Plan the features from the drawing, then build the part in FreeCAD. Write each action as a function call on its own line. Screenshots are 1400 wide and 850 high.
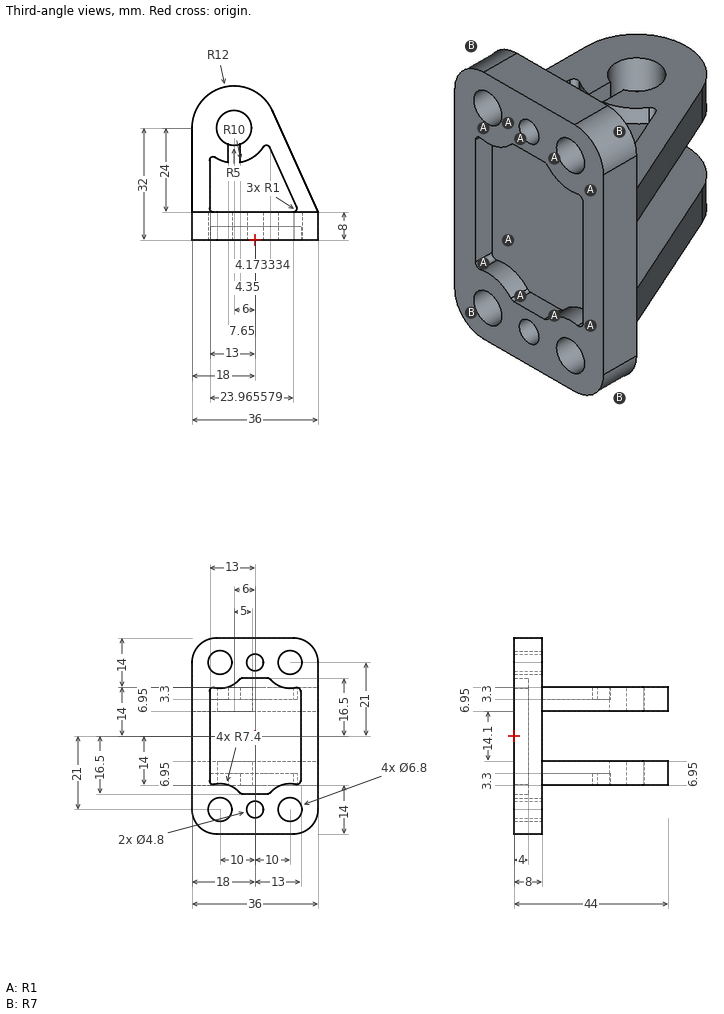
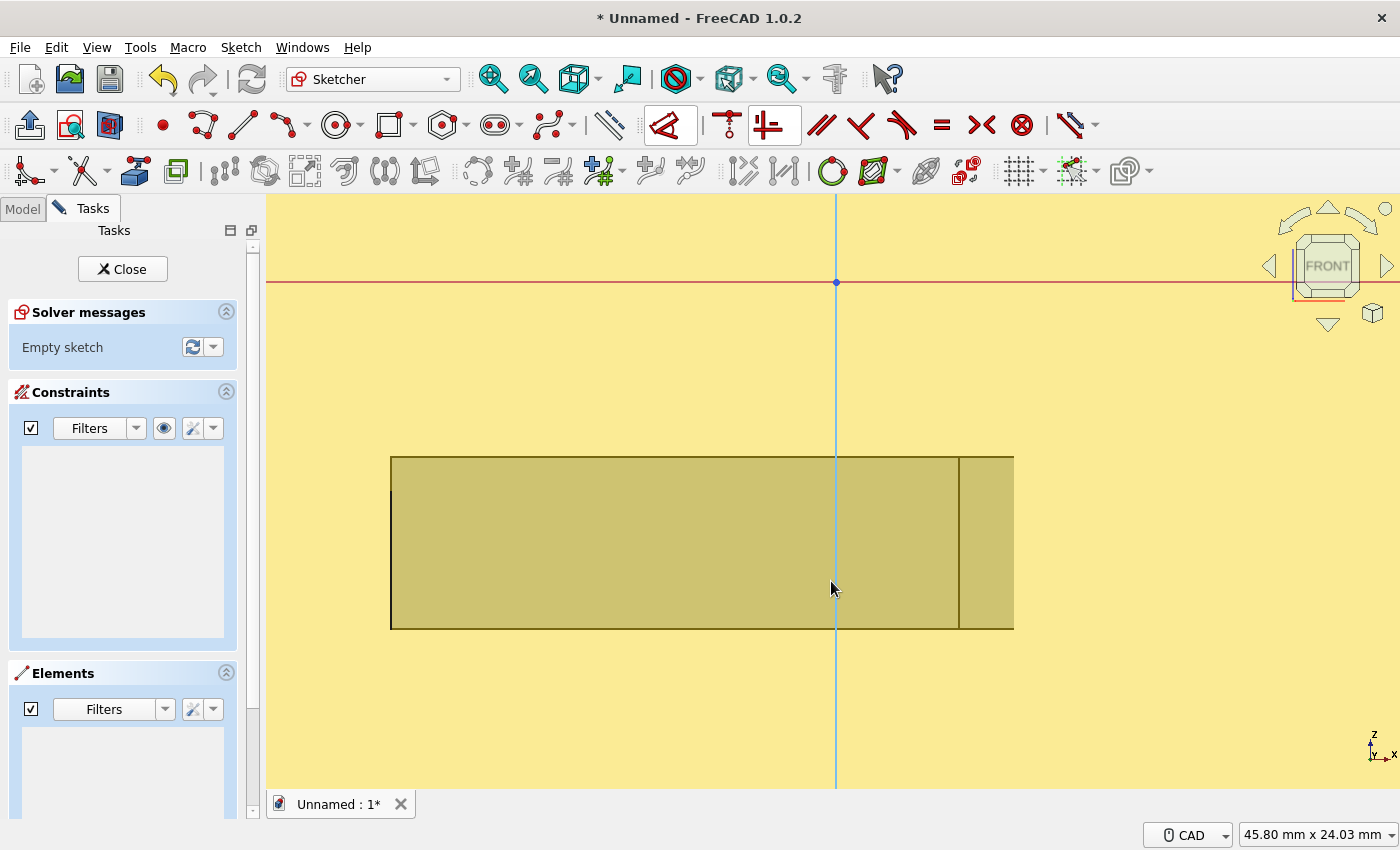
key(g)
key(r)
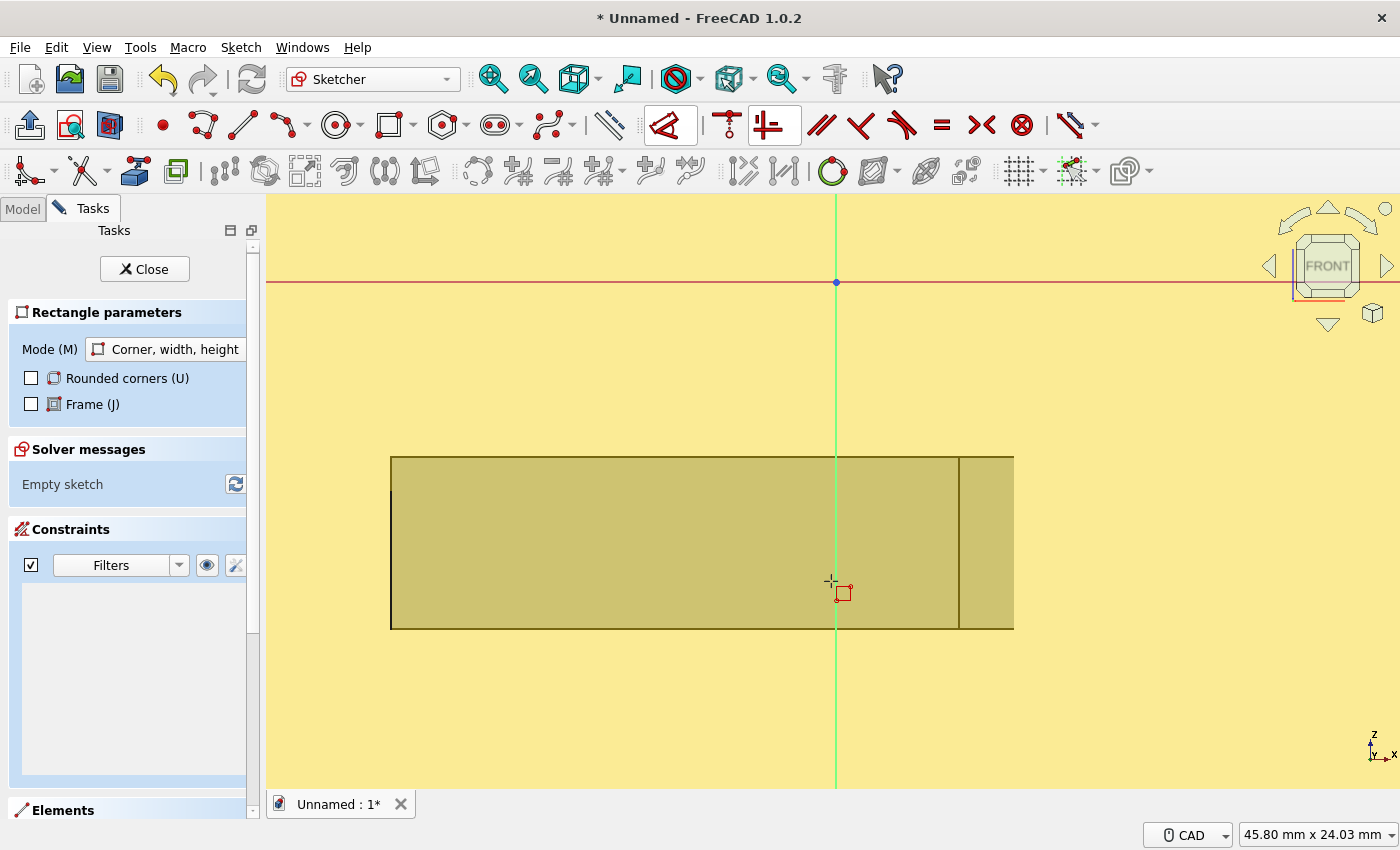
click(688, 457)
move(812, 629)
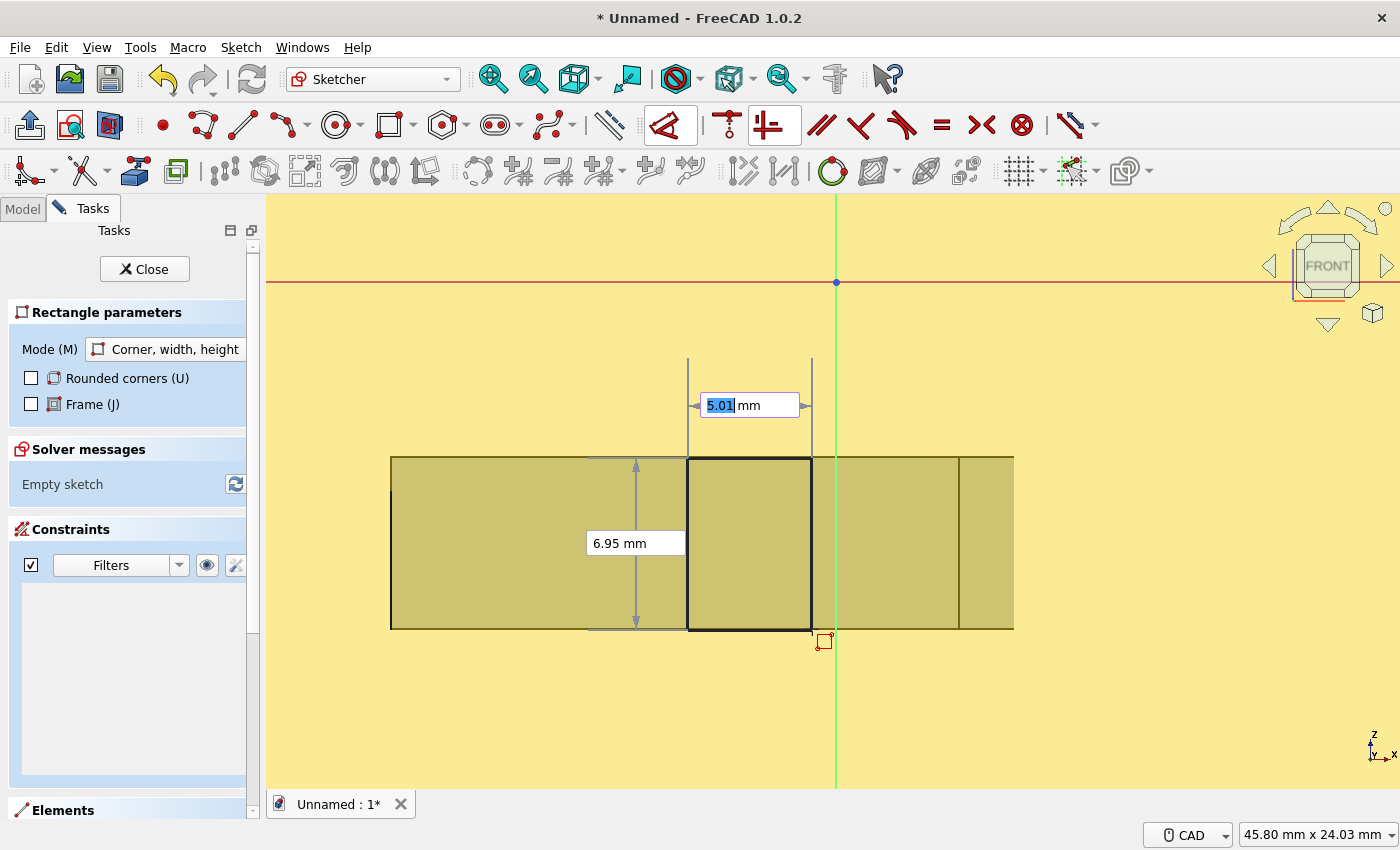
text(5)
key(Tab)
text(6.95)
key(Return)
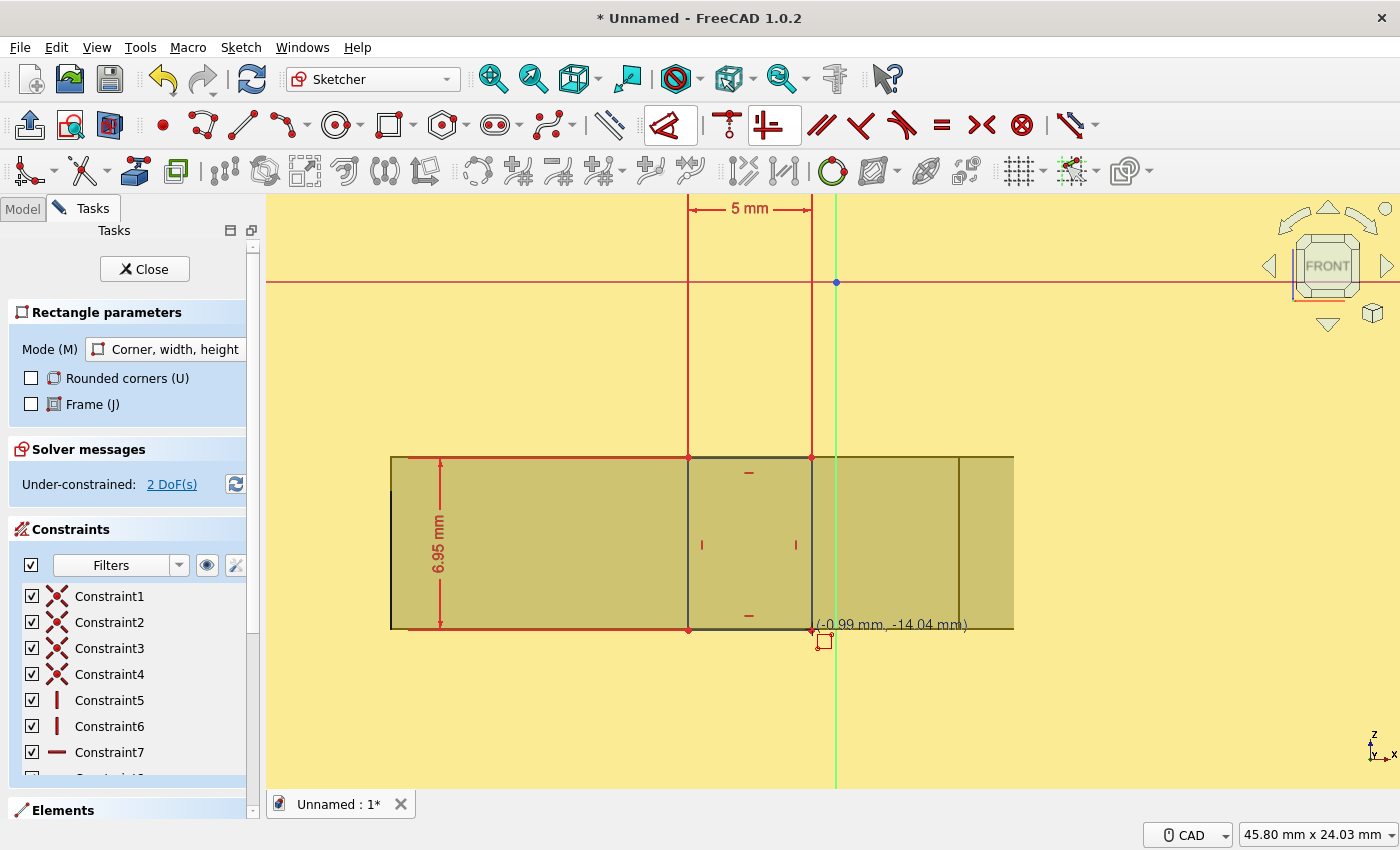
click(244, 126)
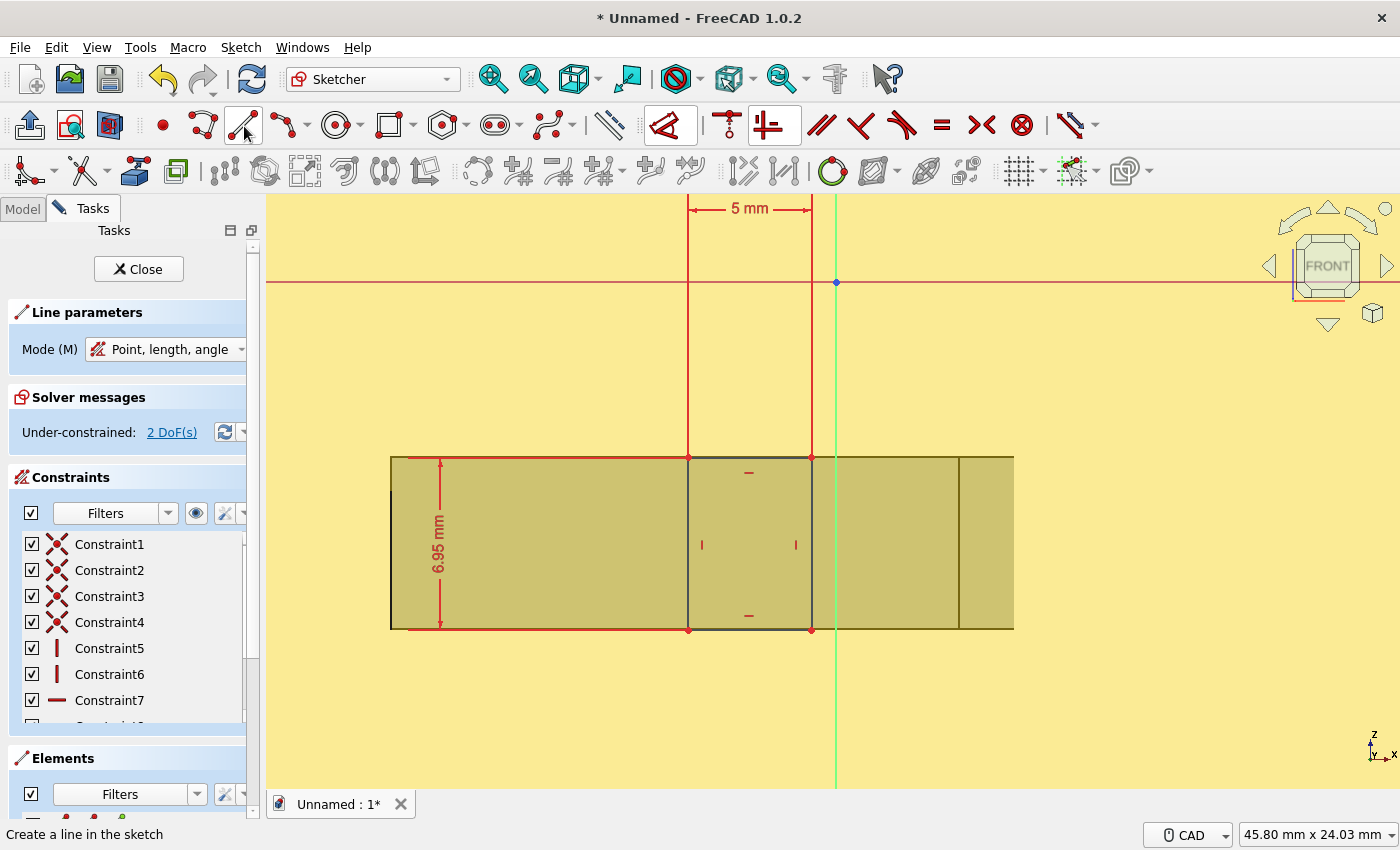
click(688, 646)
click(688, 698)
key(Escape)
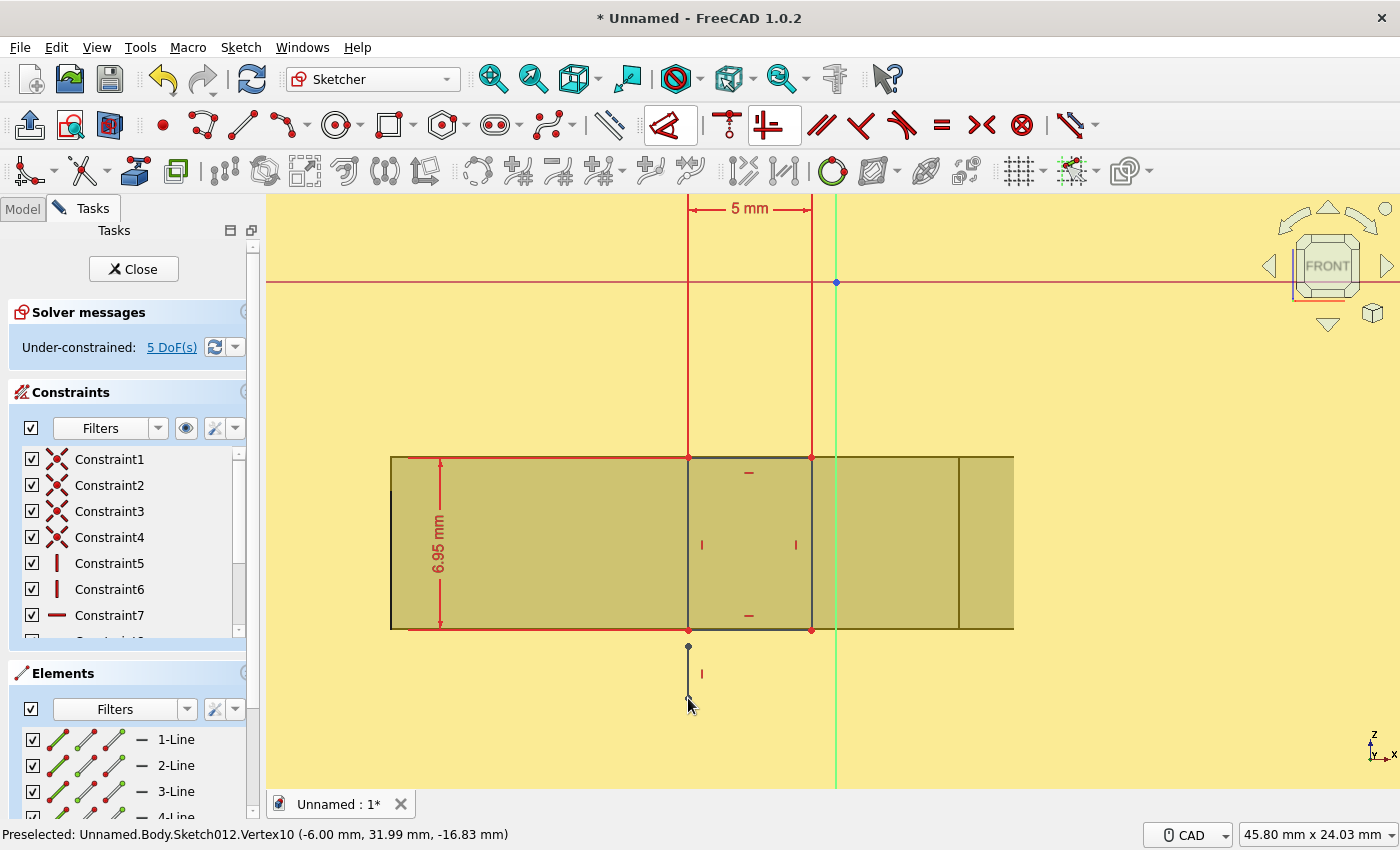
click(688, 663)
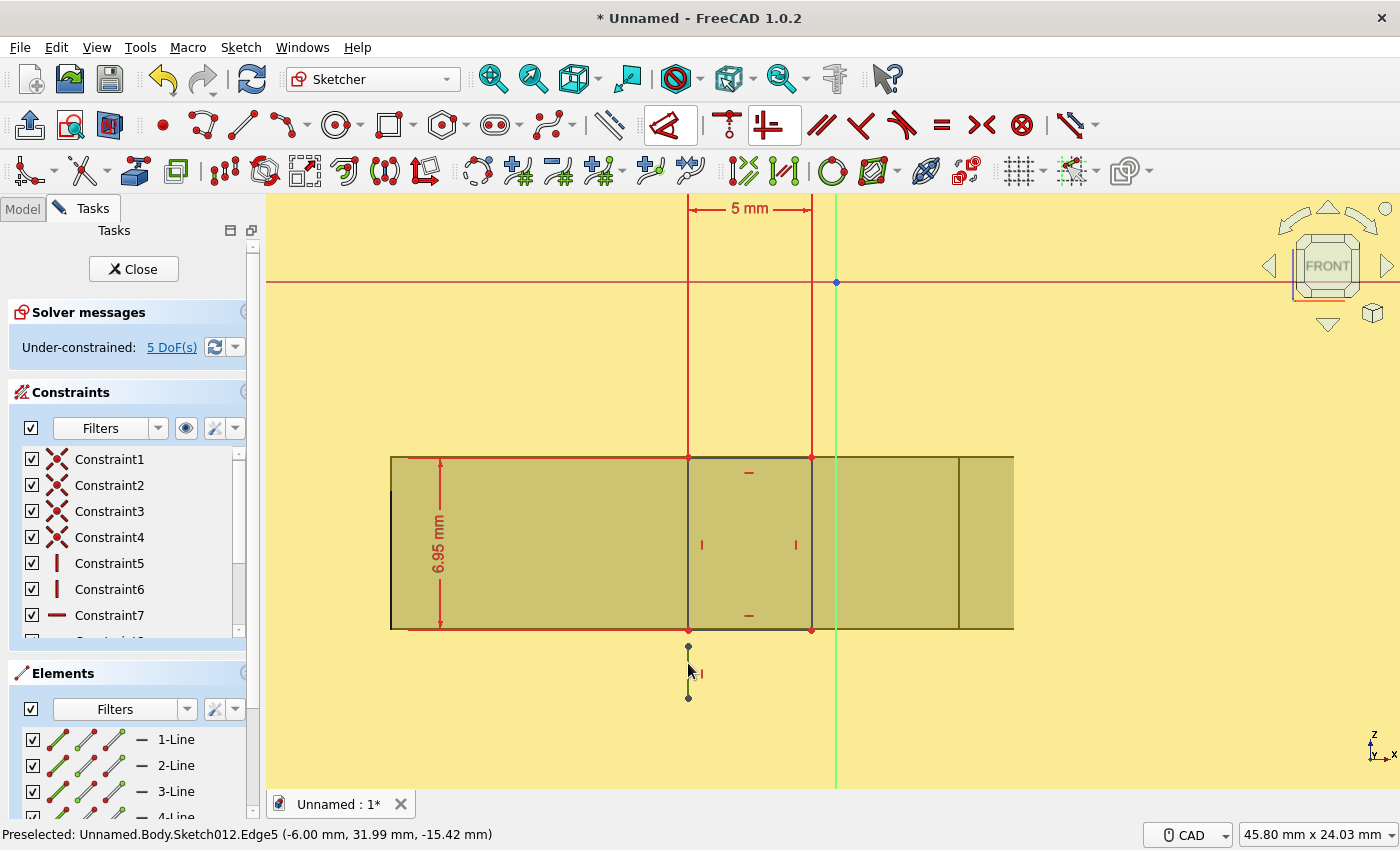
click(610, 126)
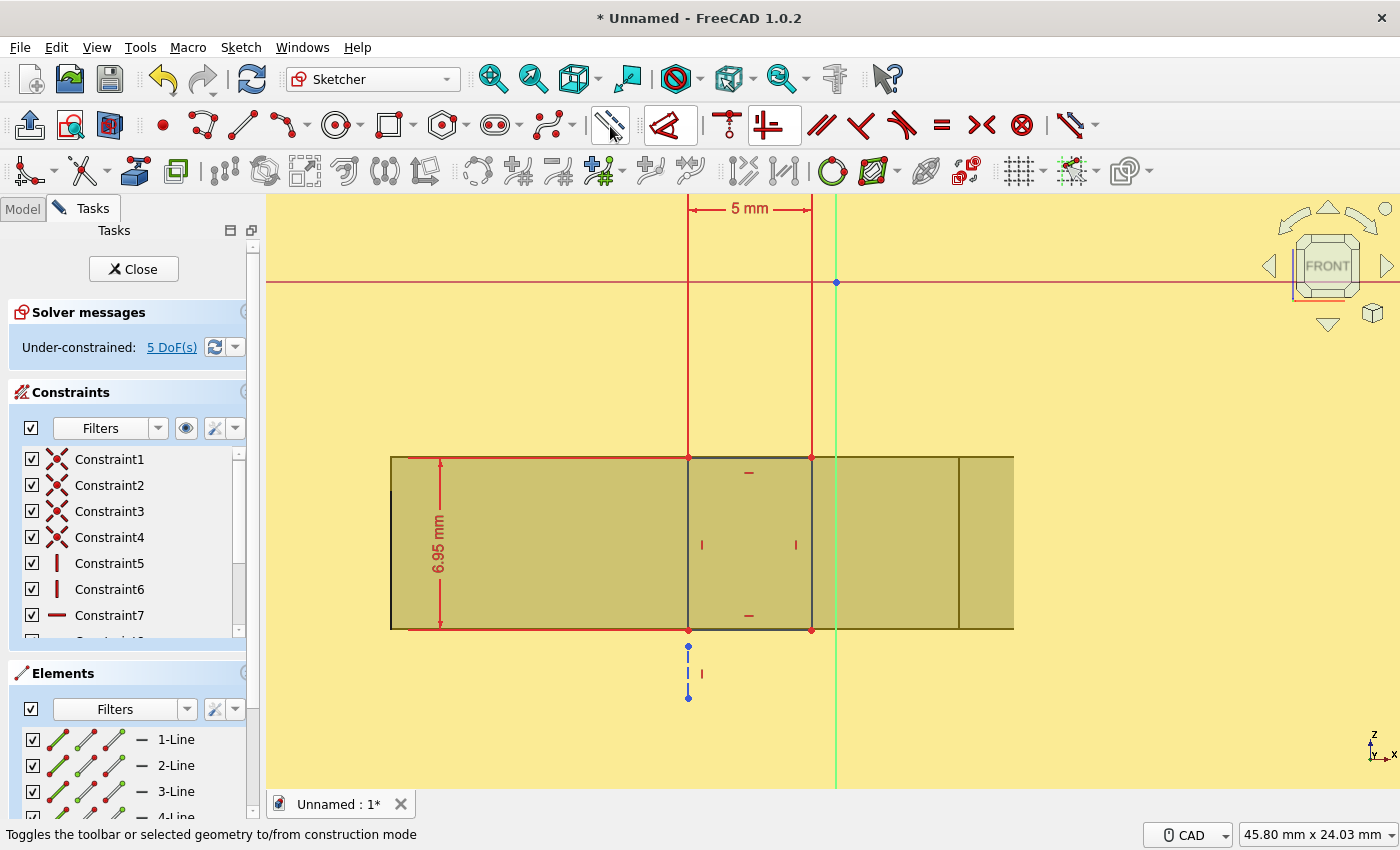
click(688, 458)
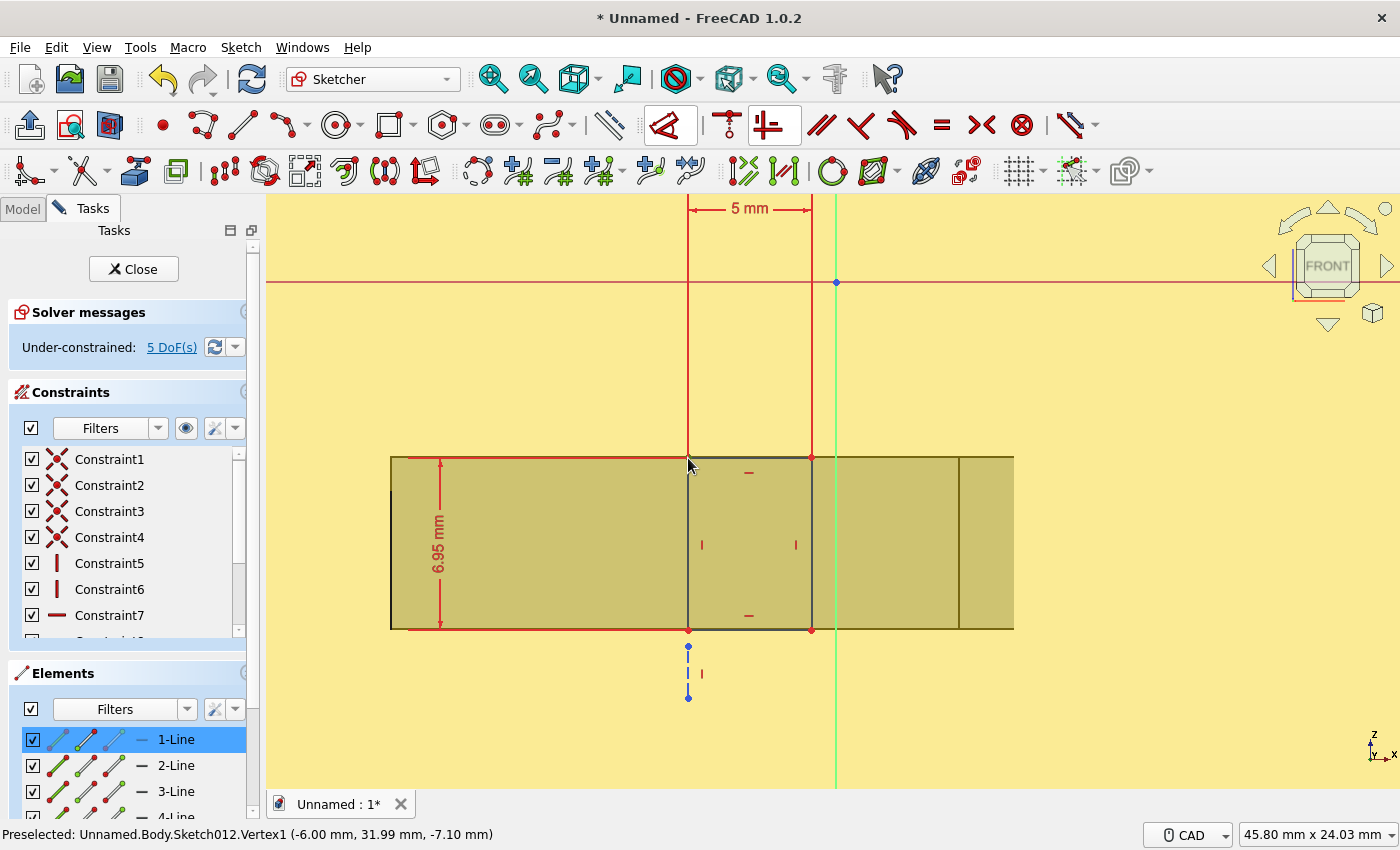
key(l)